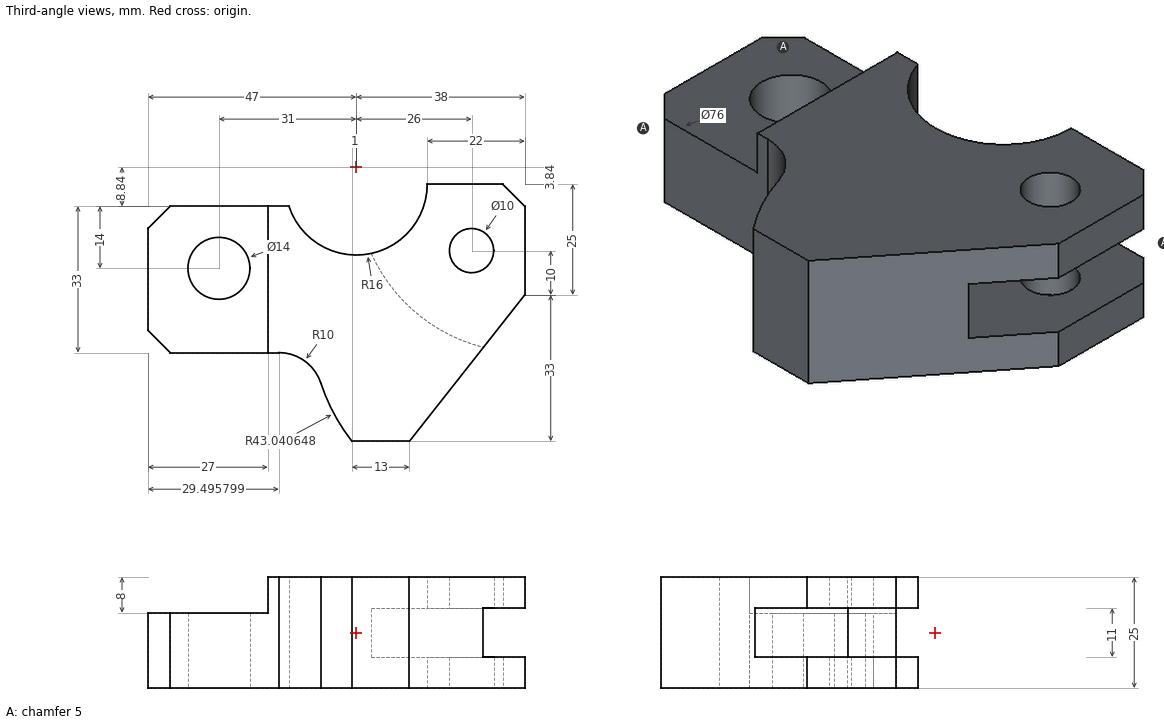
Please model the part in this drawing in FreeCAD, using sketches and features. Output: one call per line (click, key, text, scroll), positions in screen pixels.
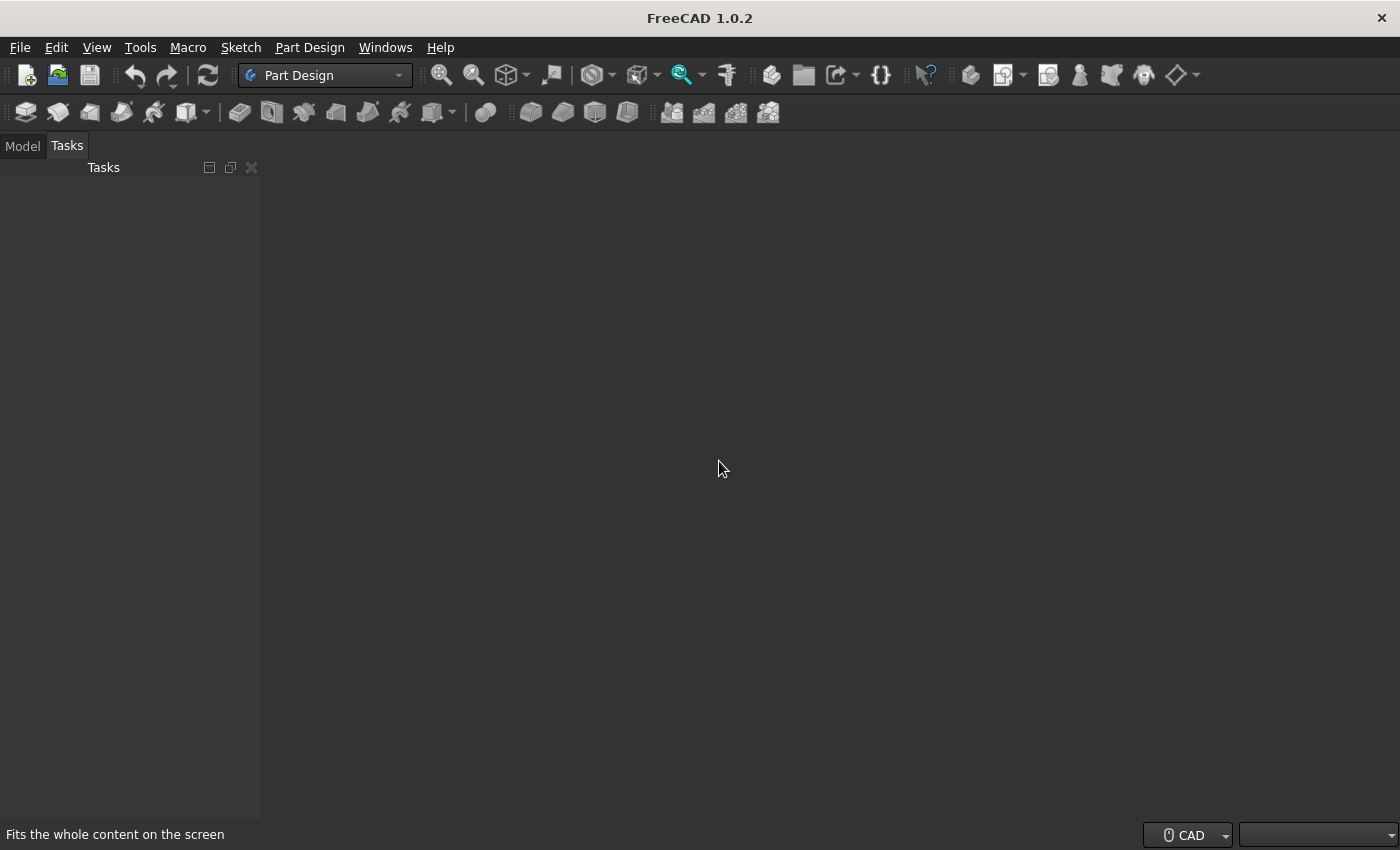
click(26, 76)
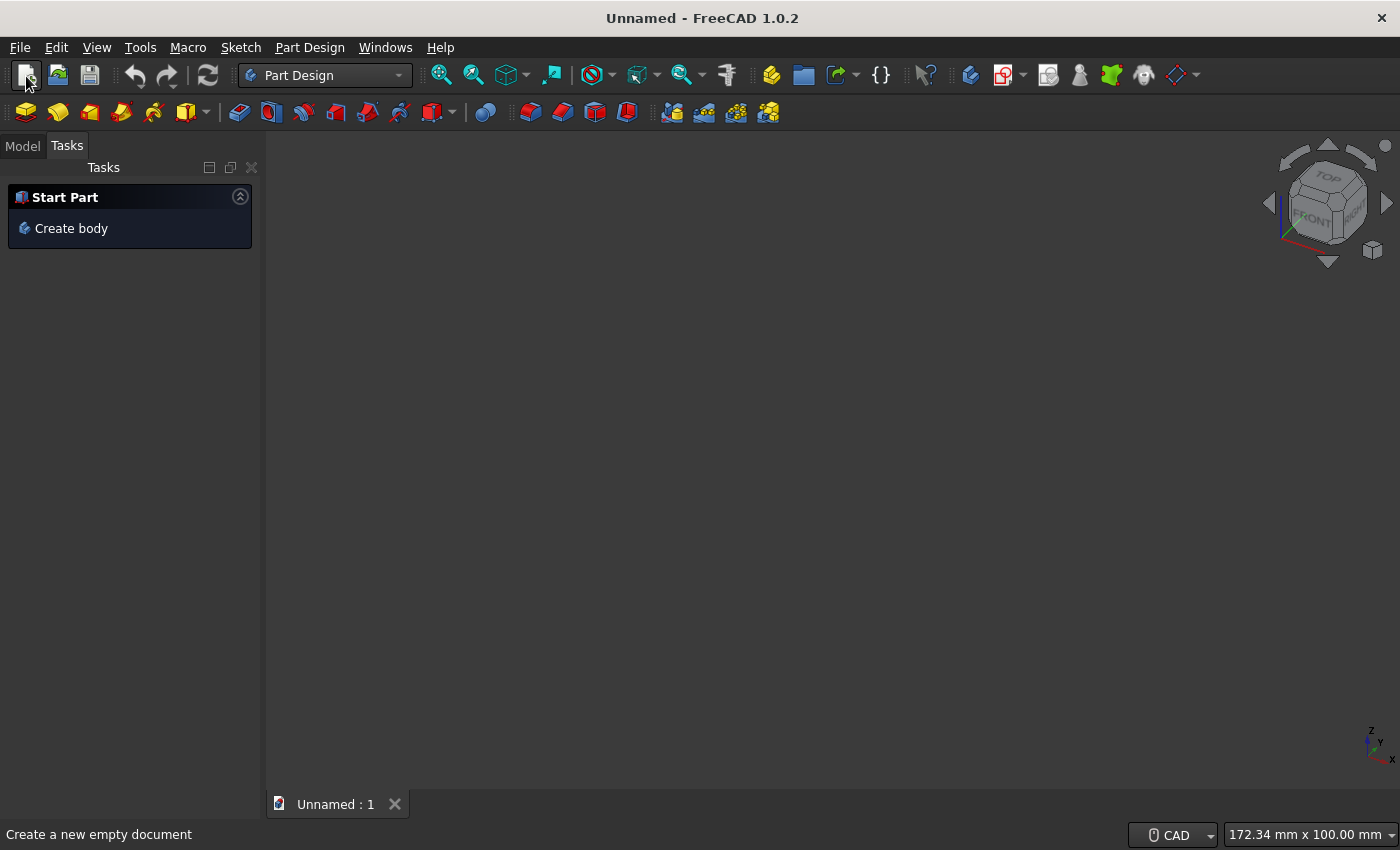
click(1004, 76)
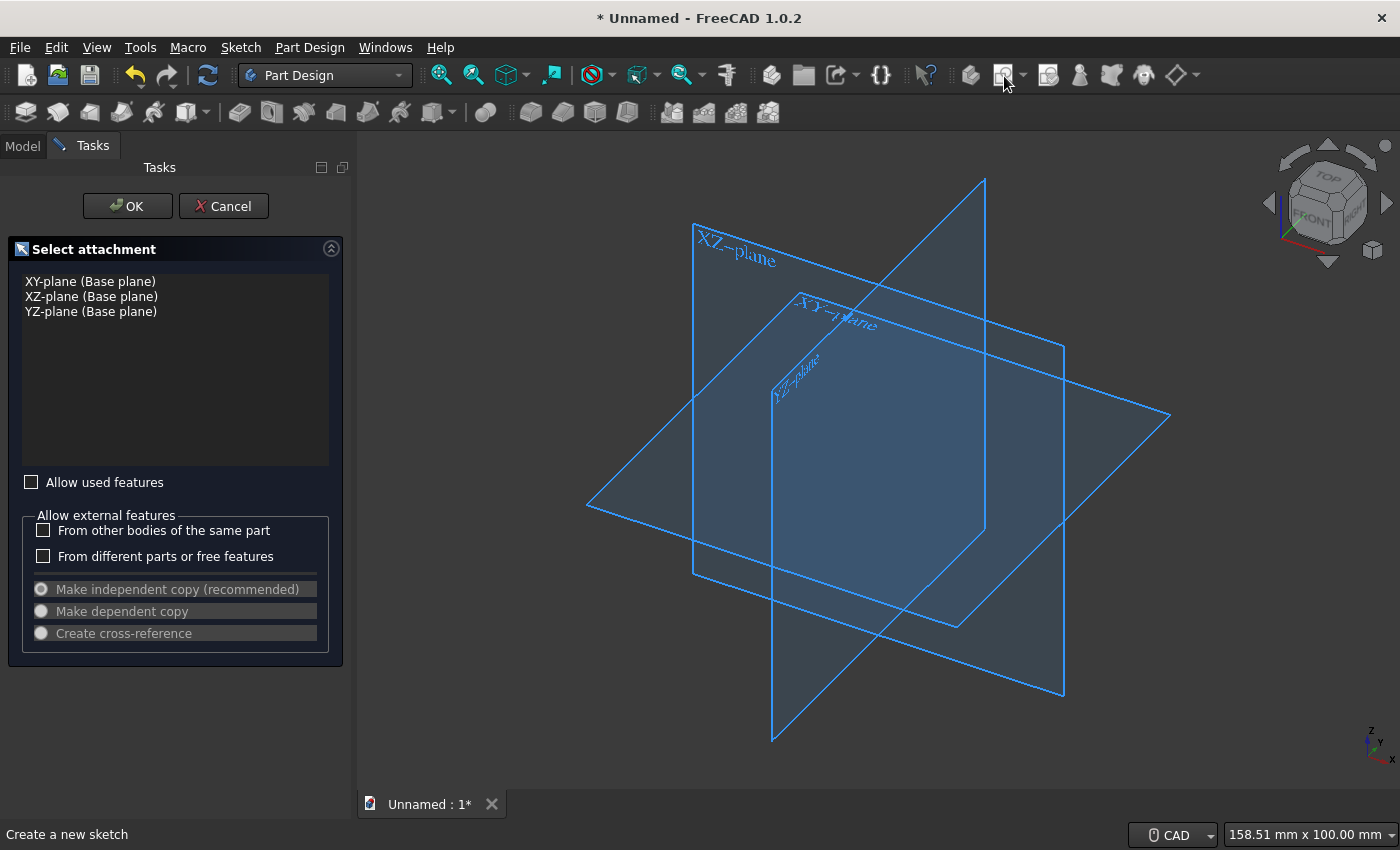
click(82, 282)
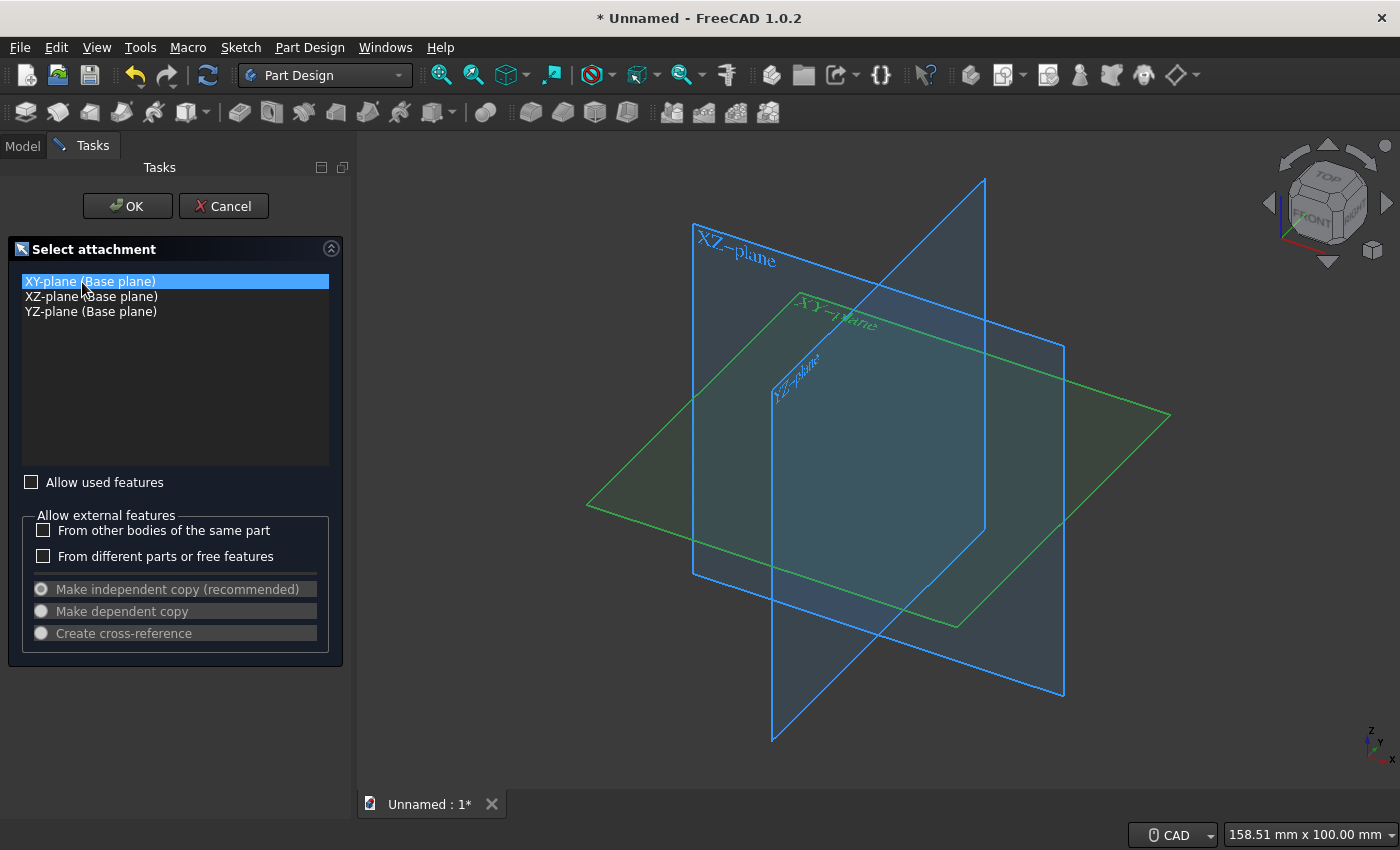
click(128, 206)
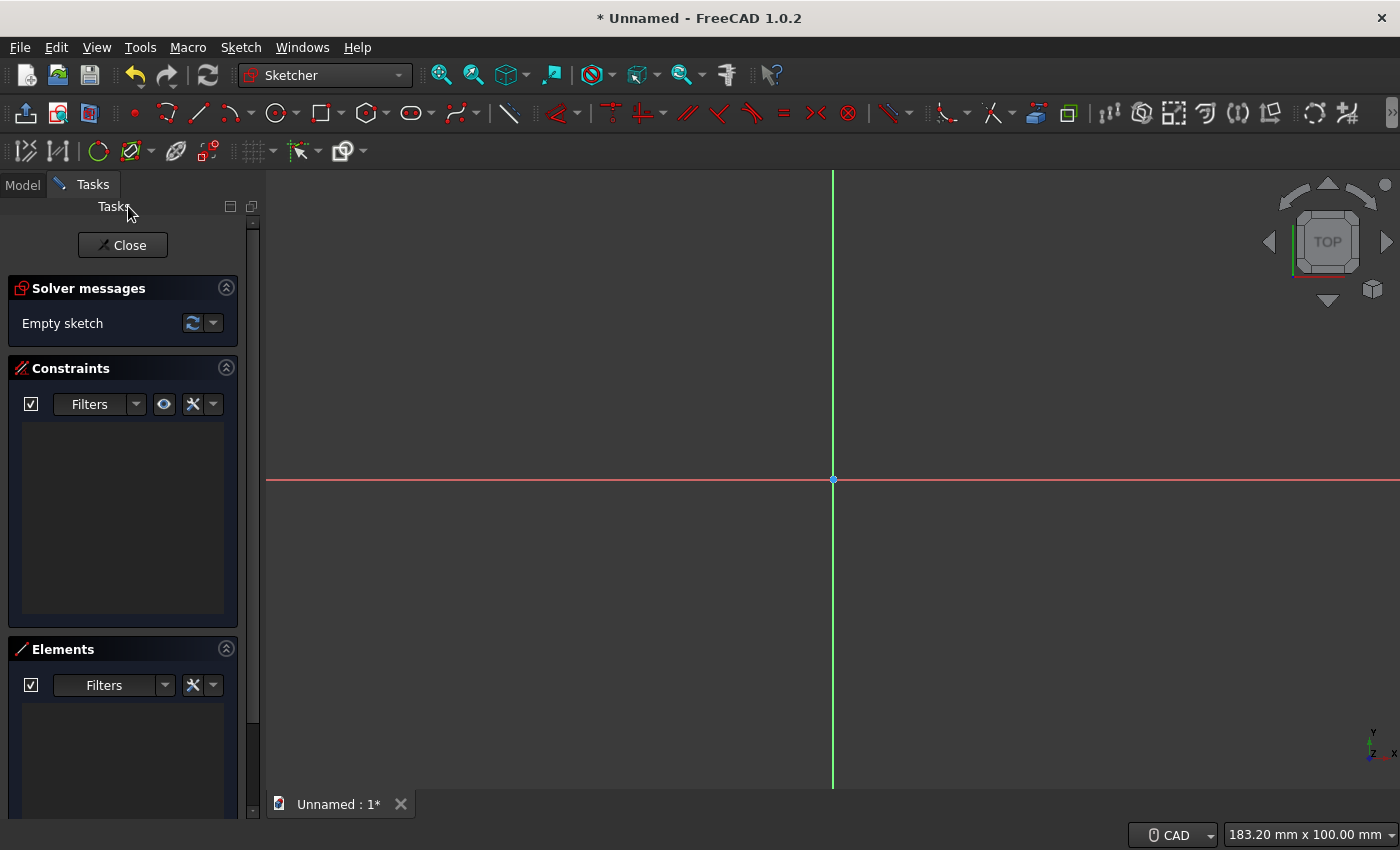
scroll(682, 198, down, 2)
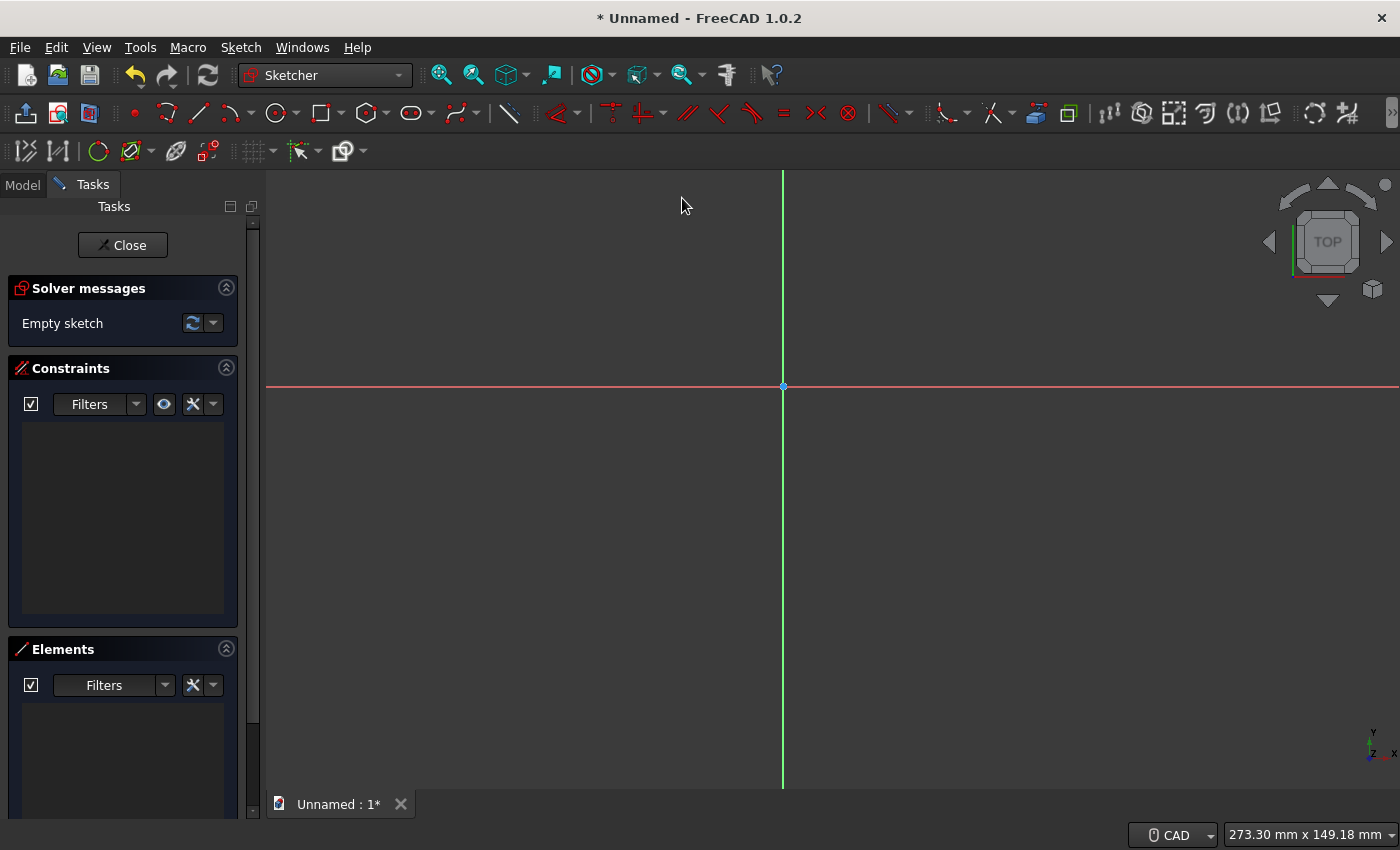
scroll(765, 587, up, 2)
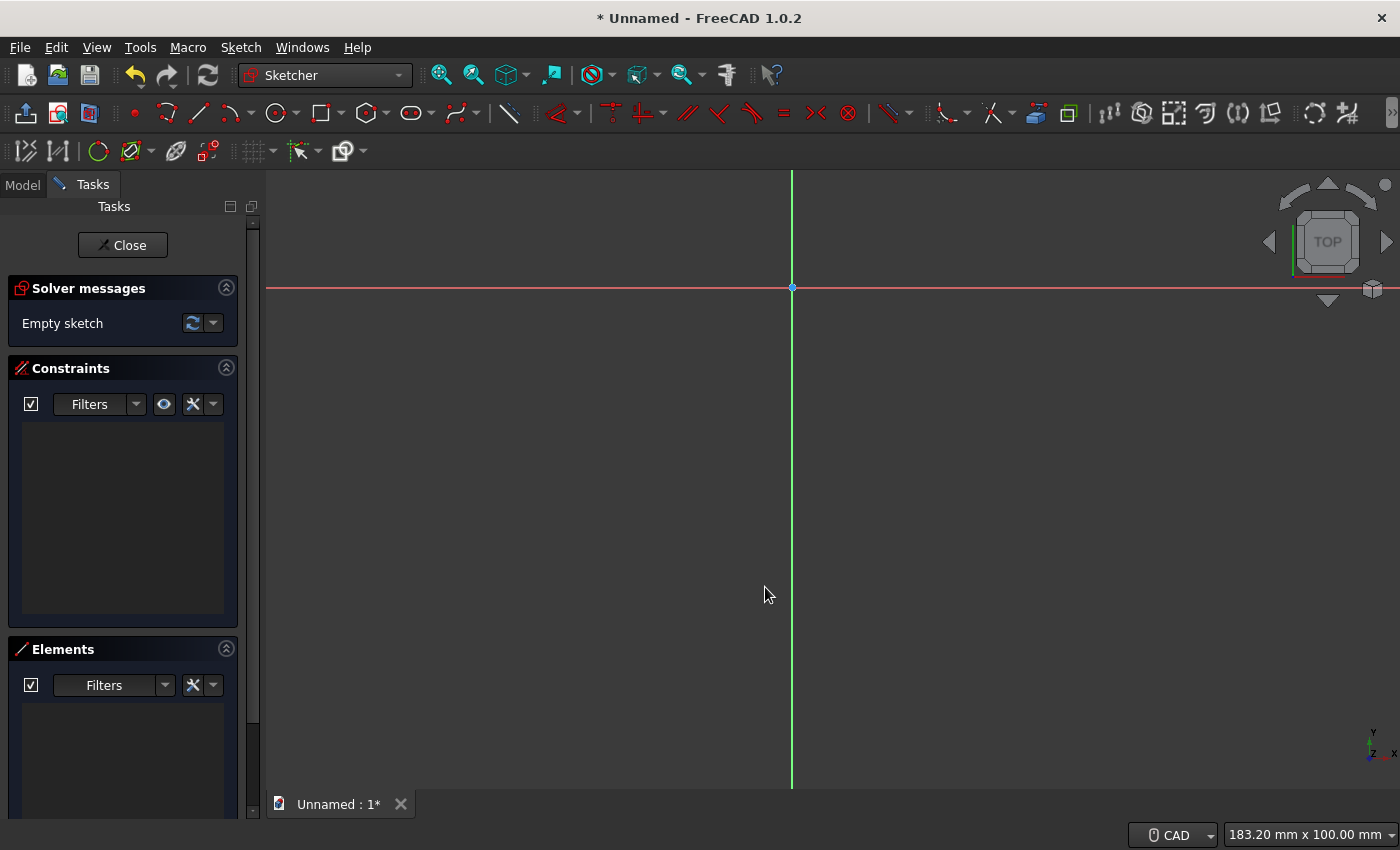
key(g)
key(m)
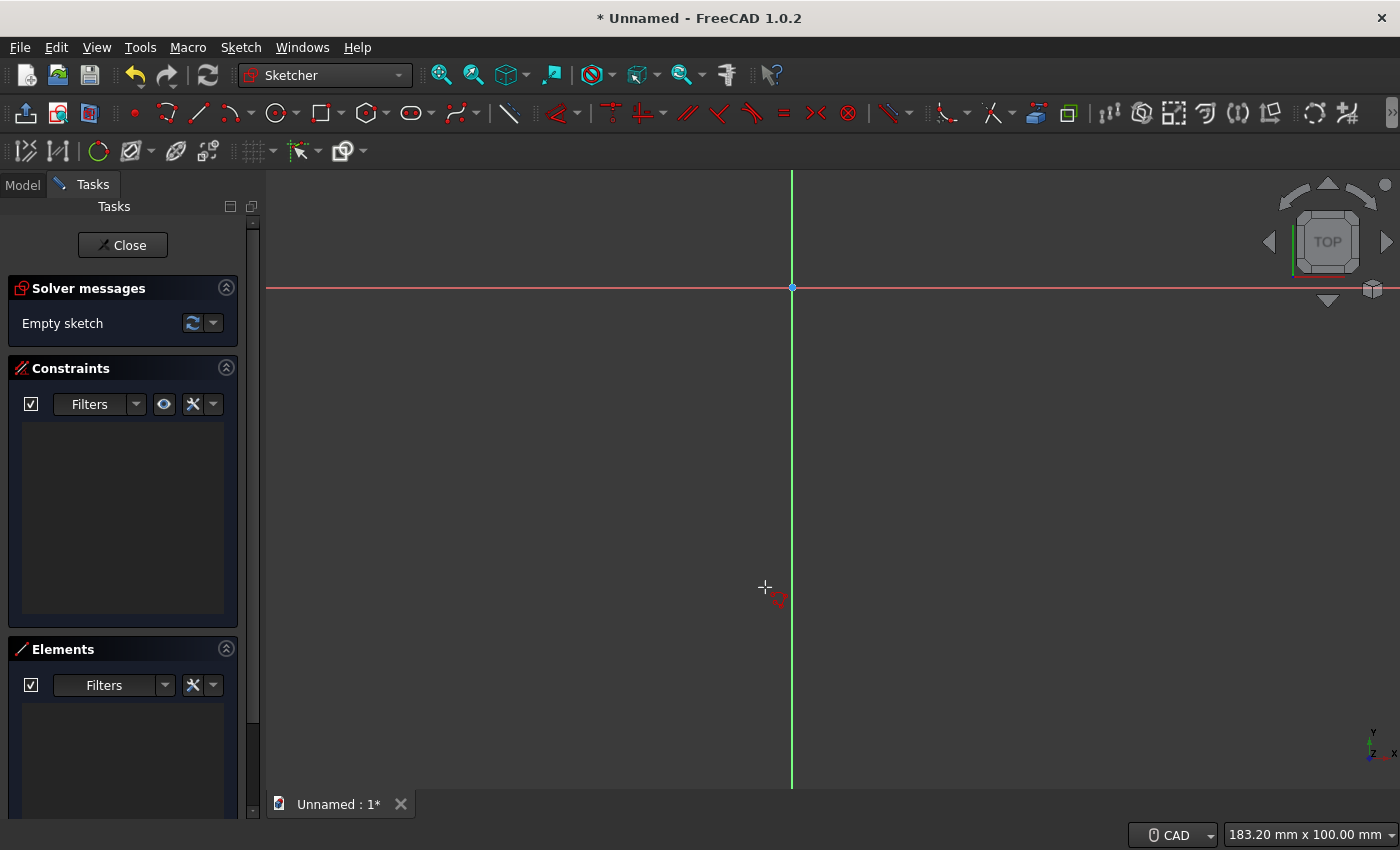
click(698, 343)
click(501, 343)
click(501, 547)
click(684, 547)
right_click(684, 547)